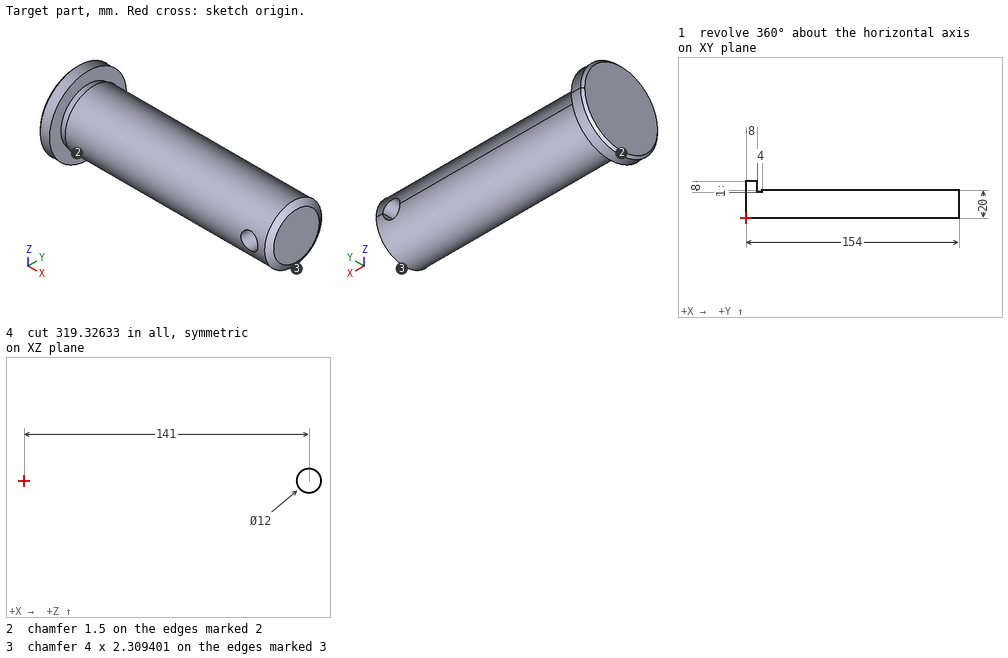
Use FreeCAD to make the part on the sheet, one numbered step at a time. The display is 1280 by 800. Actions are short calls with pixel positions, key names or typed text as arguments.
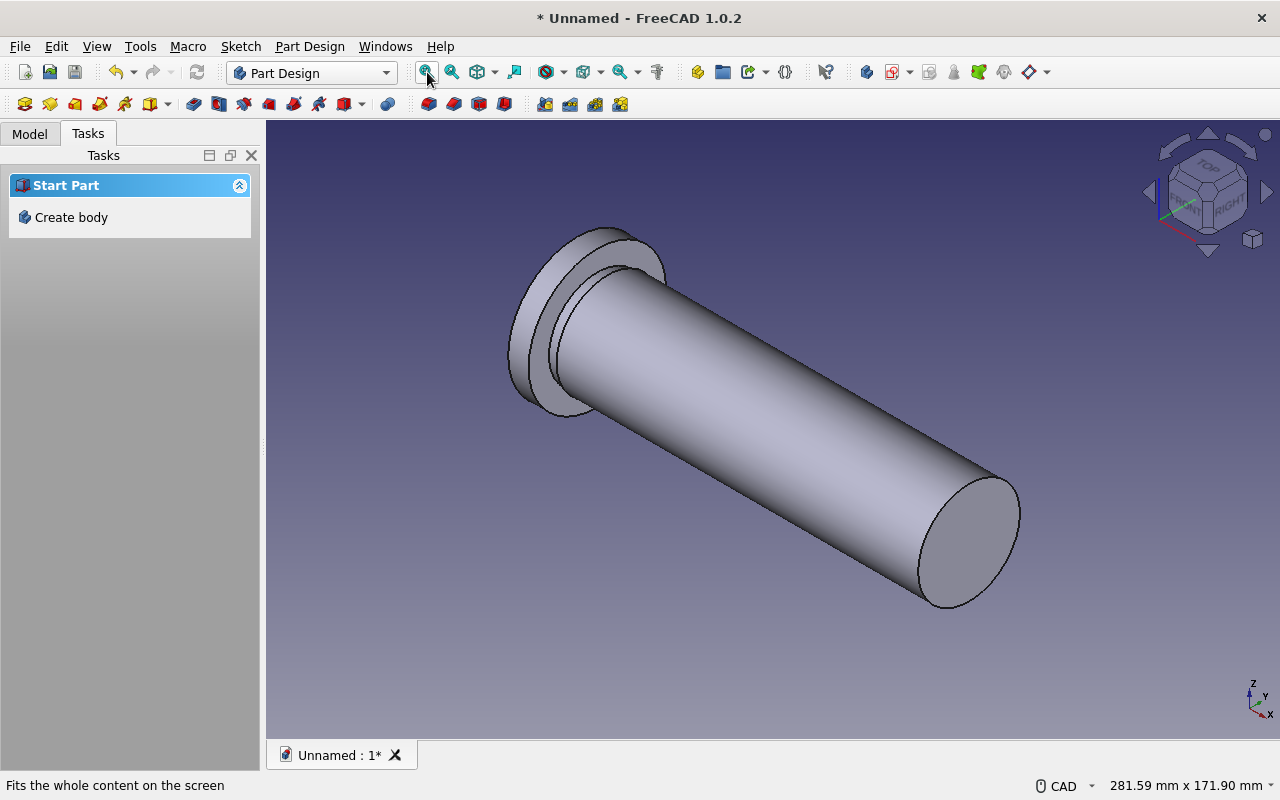
key(2)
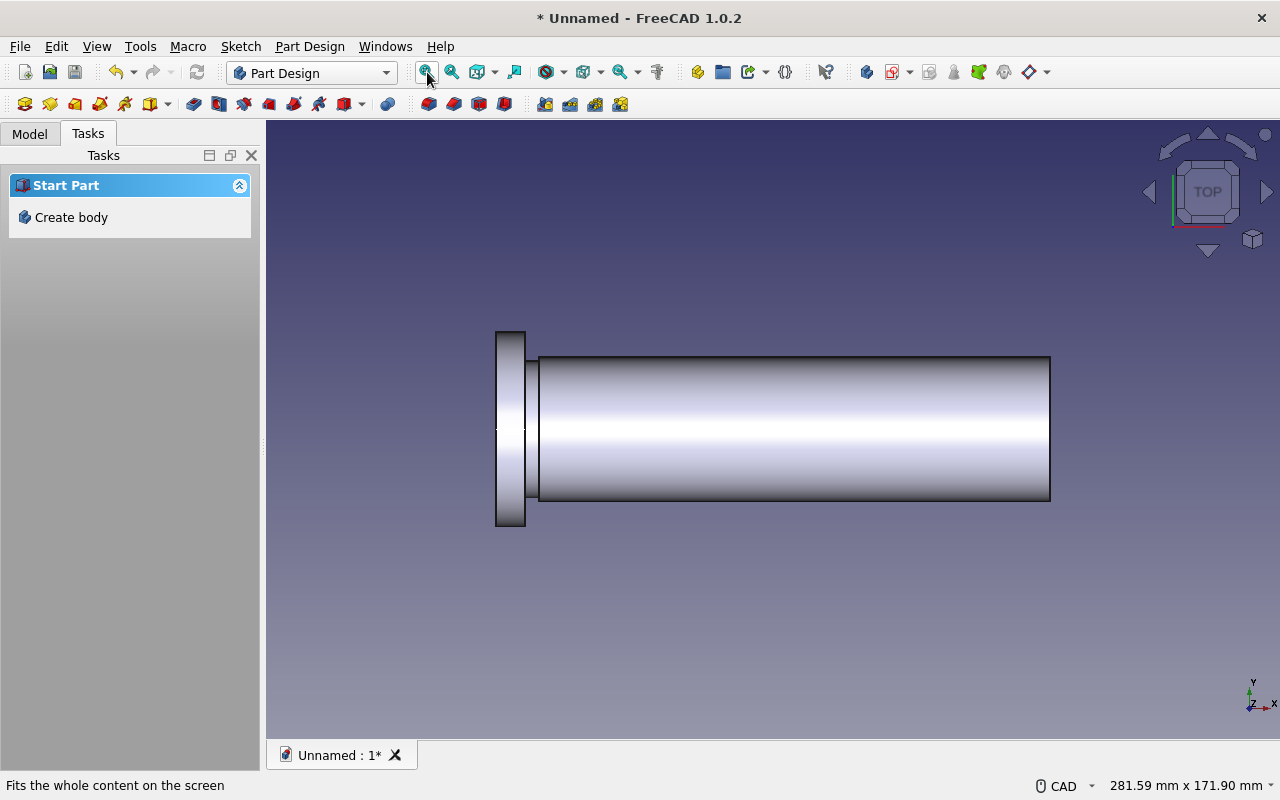
click(496, 507)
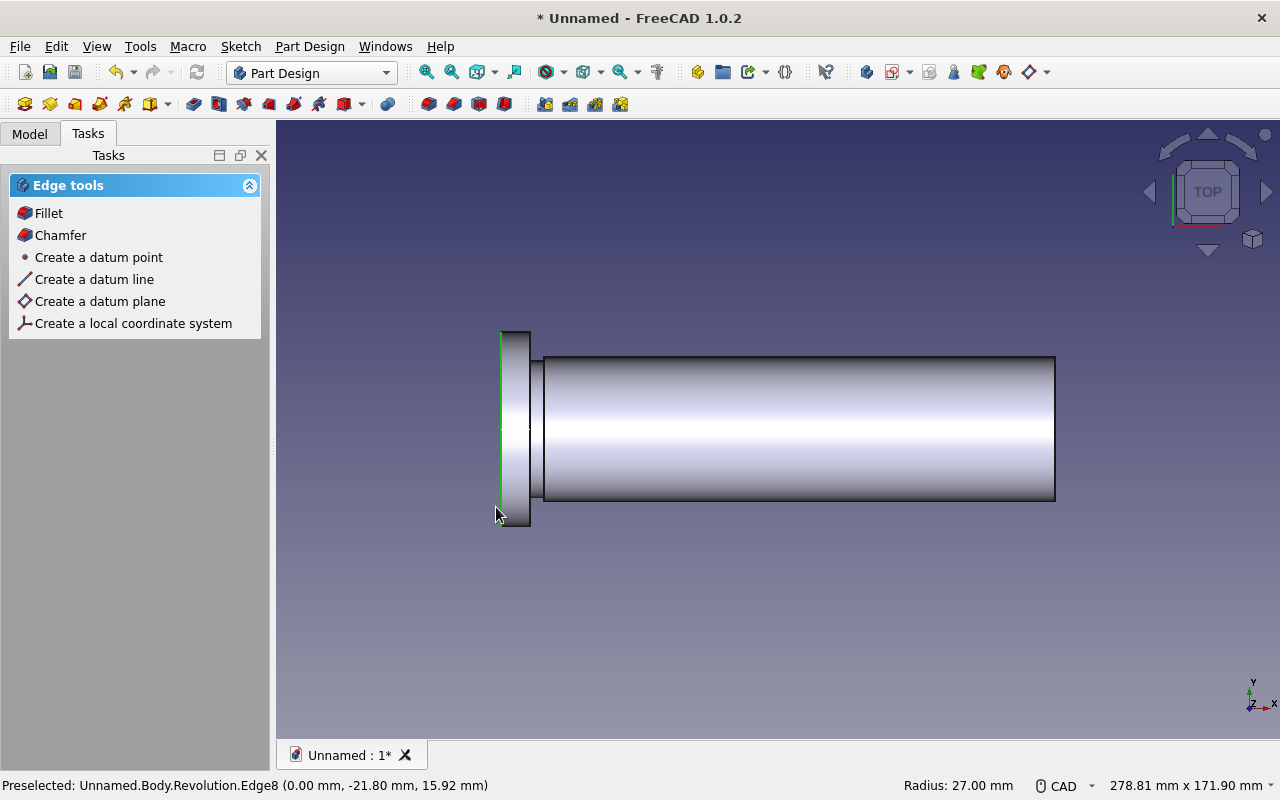
click(454, 104)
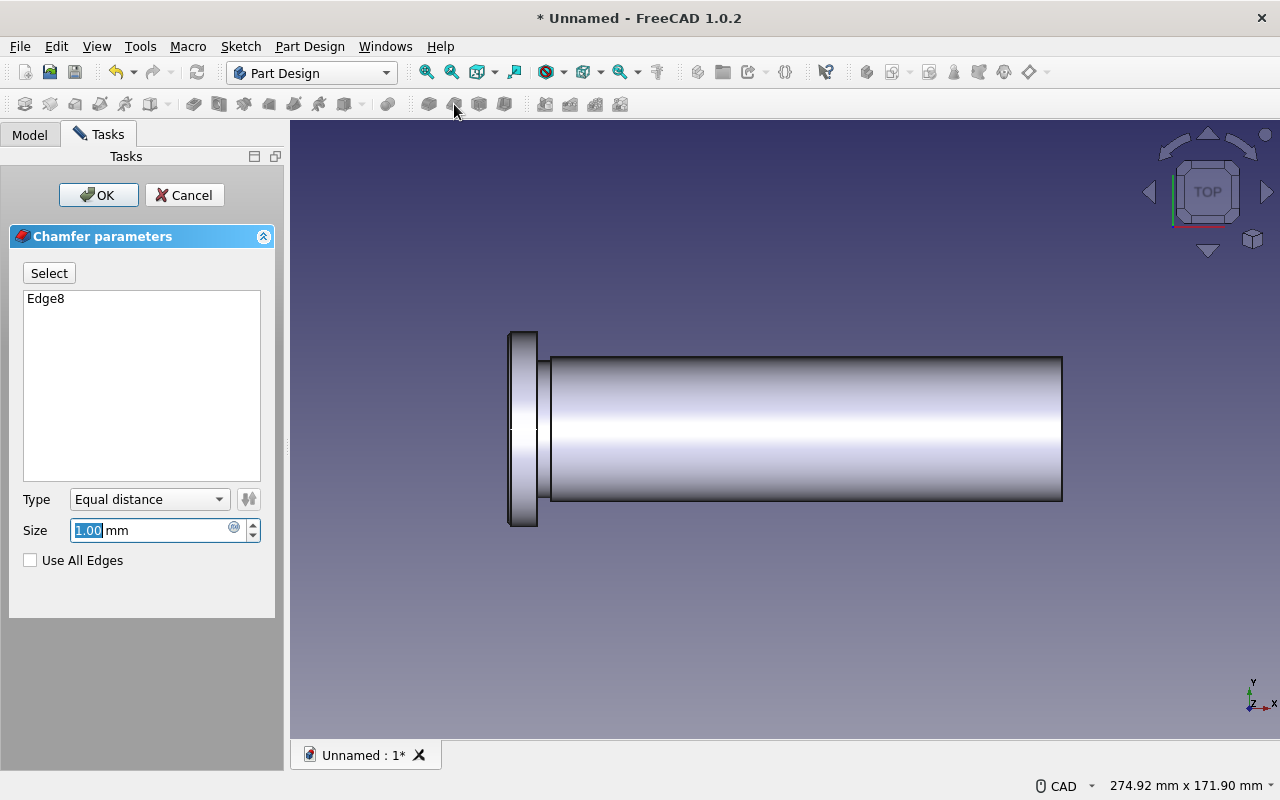
text(1.5)
key(Tab)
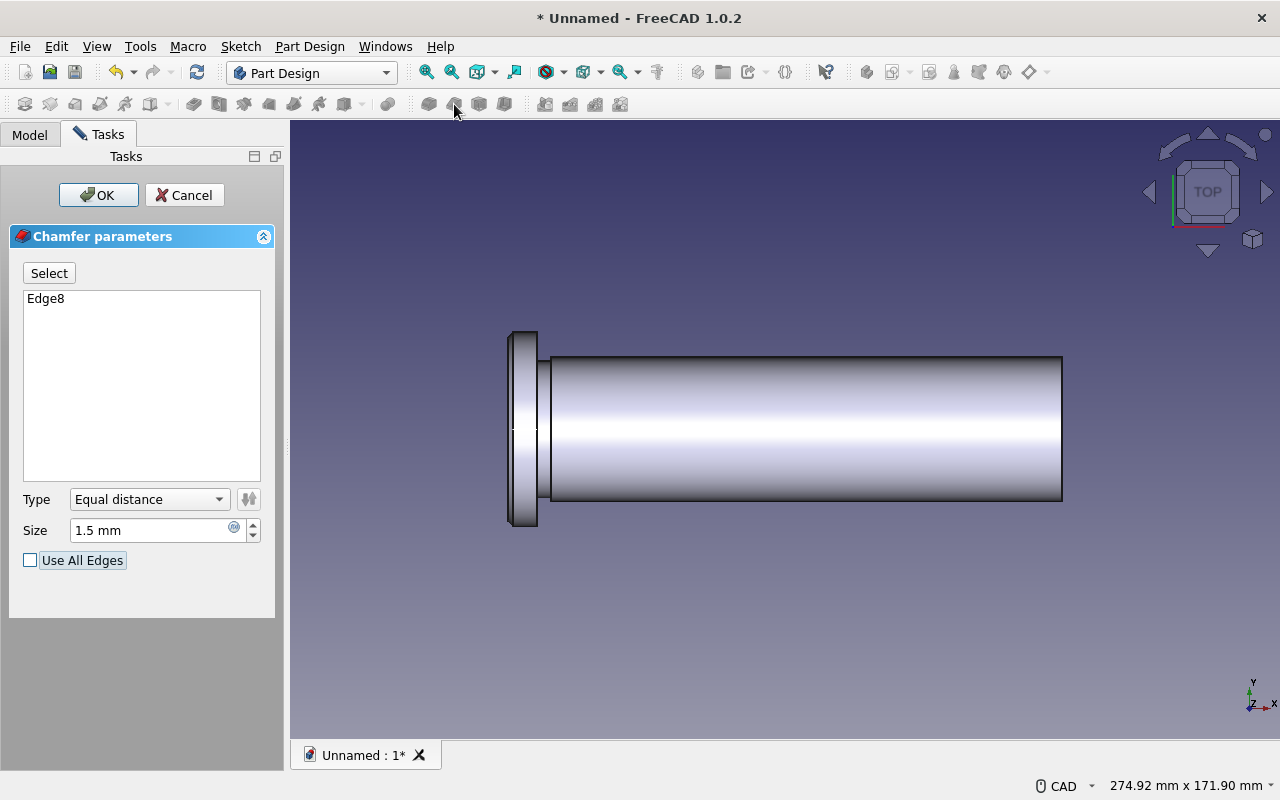
click(99, 195)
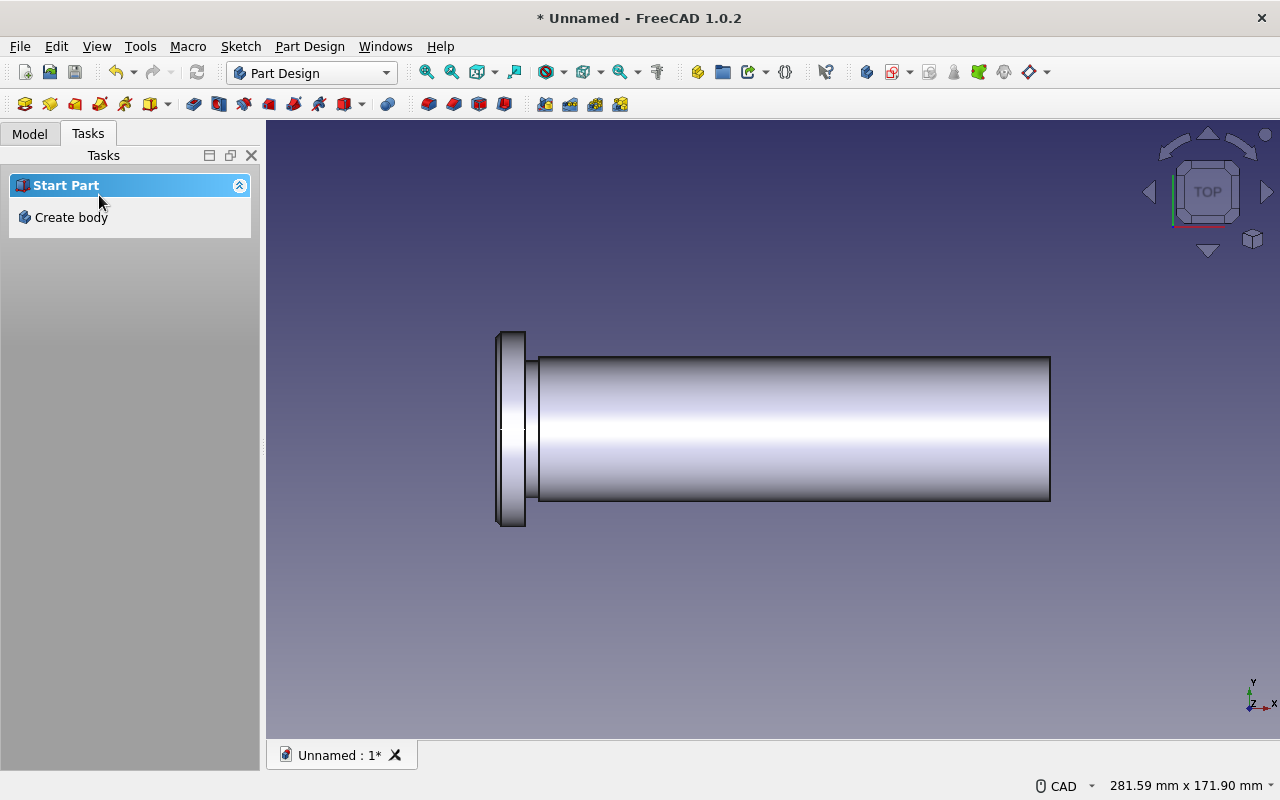
click(1050, 487)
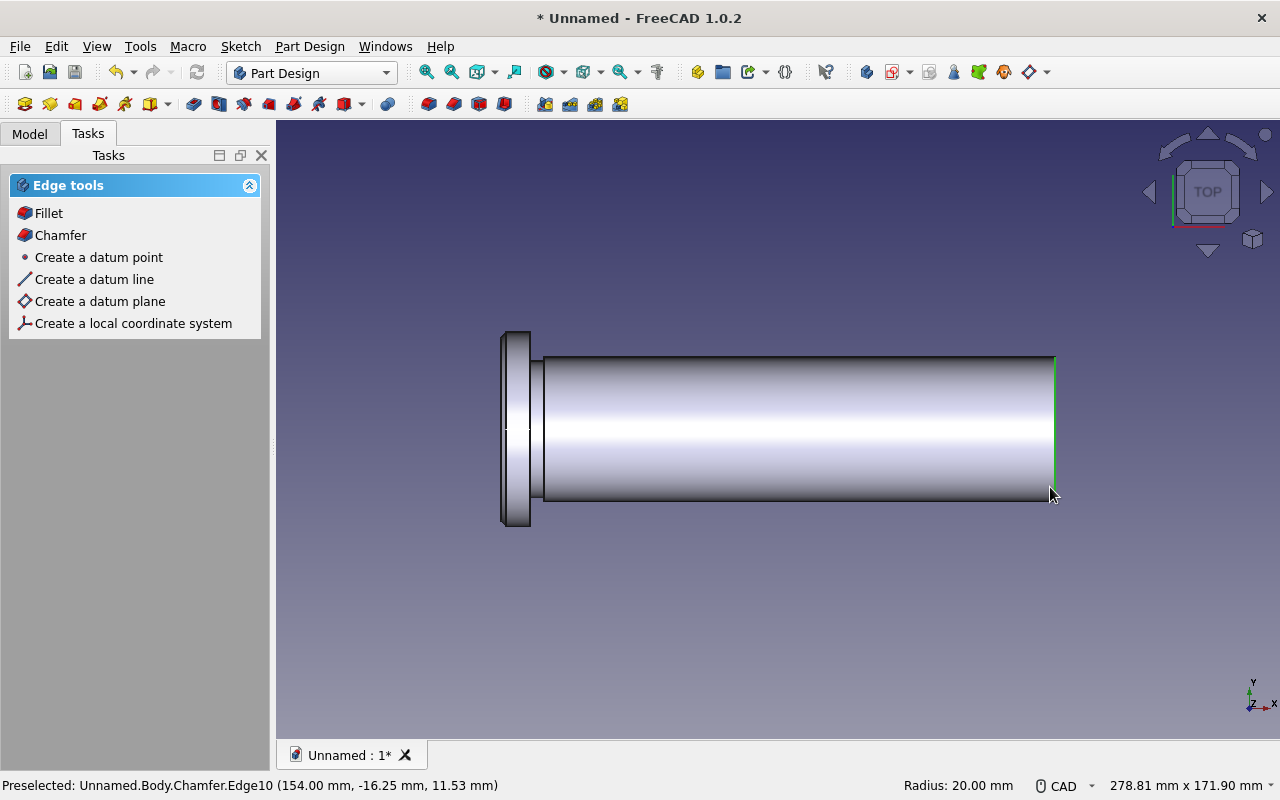
click(454, 104)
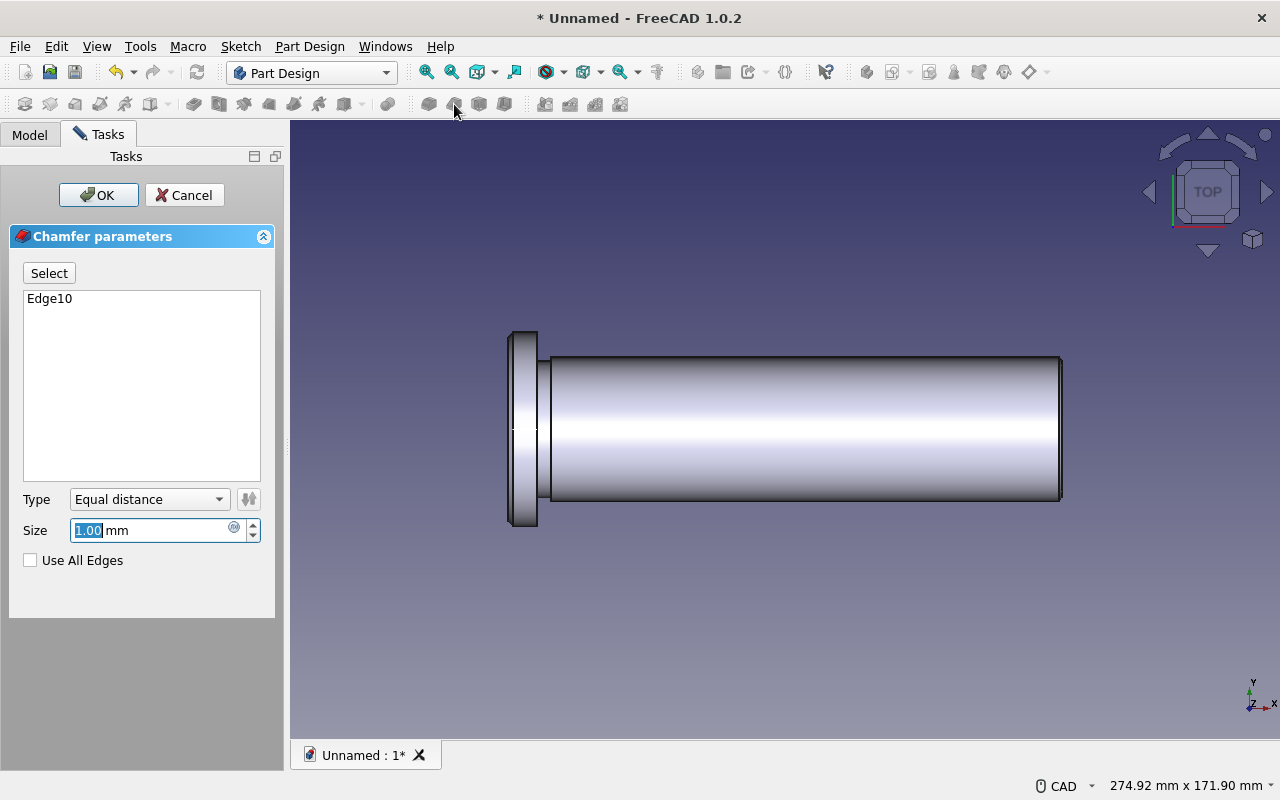
text(4)
key(Tab)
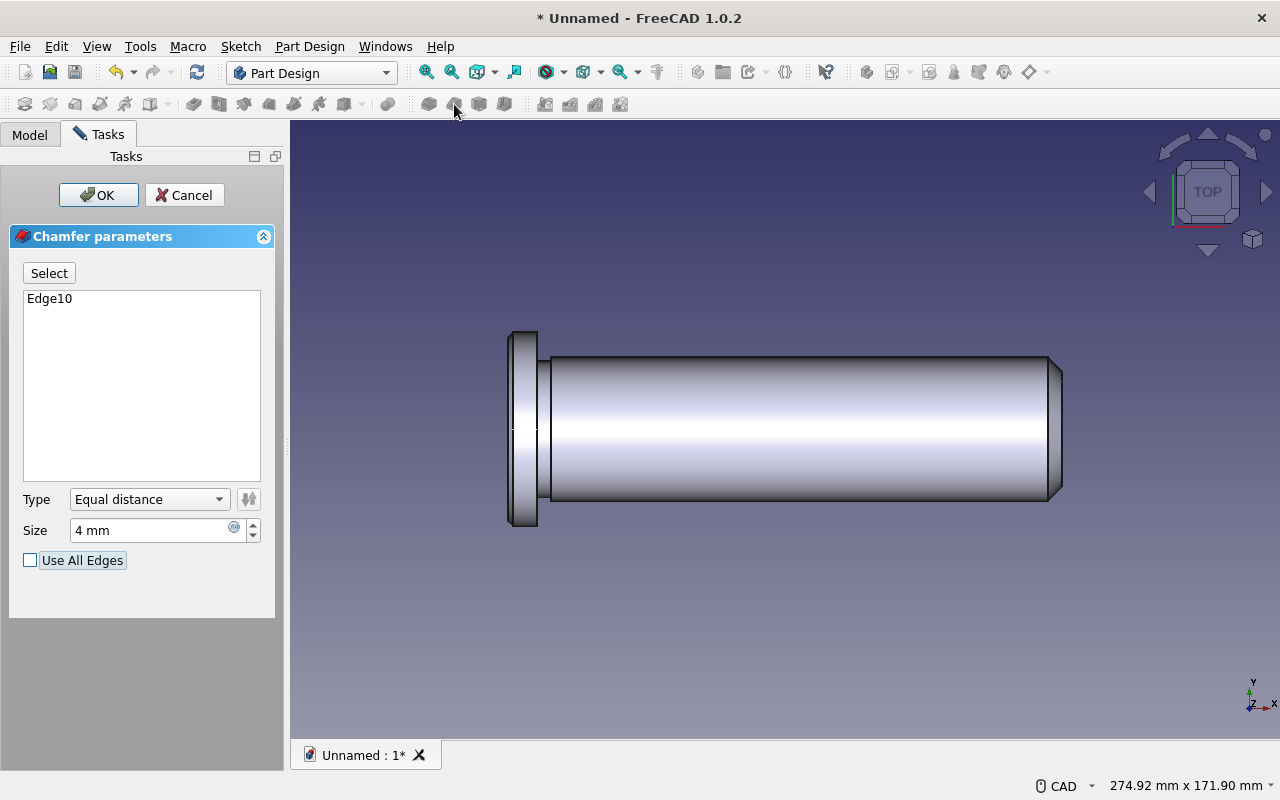
click(150, 500)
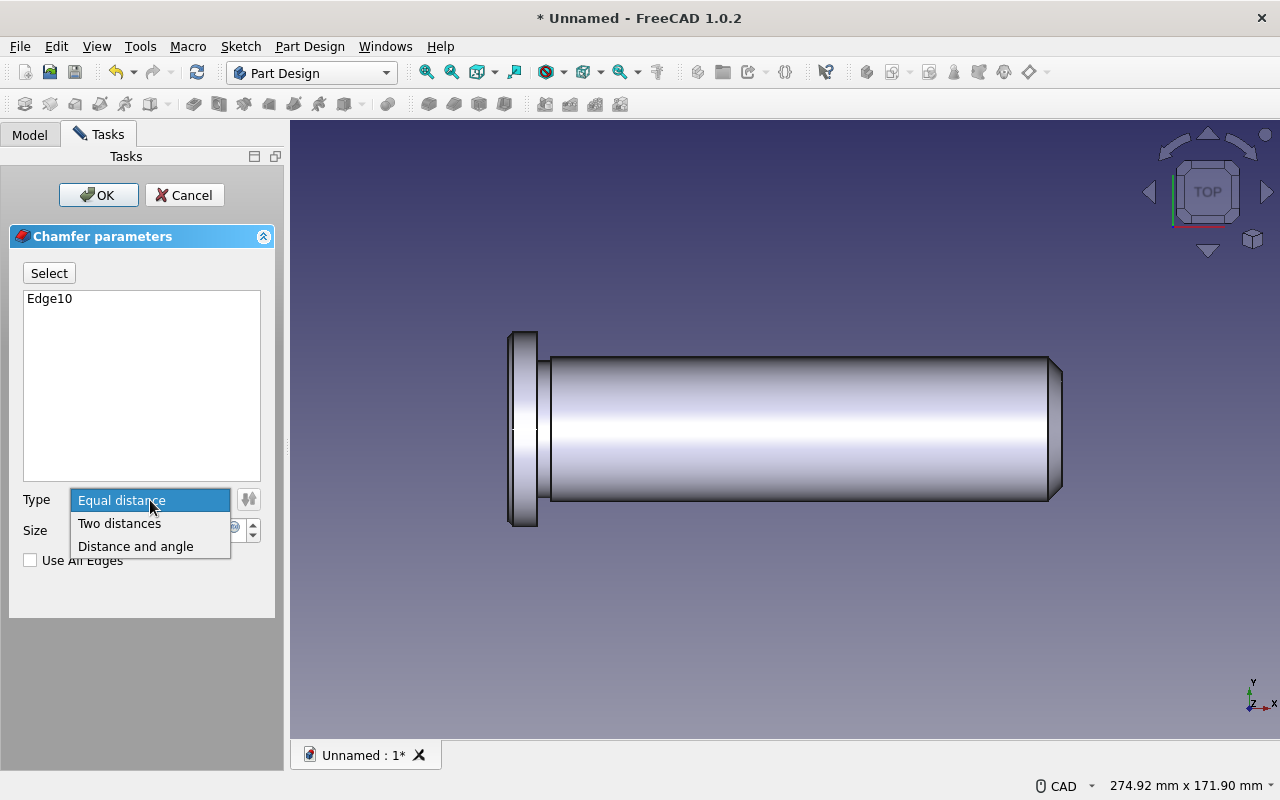
click(148, 524)